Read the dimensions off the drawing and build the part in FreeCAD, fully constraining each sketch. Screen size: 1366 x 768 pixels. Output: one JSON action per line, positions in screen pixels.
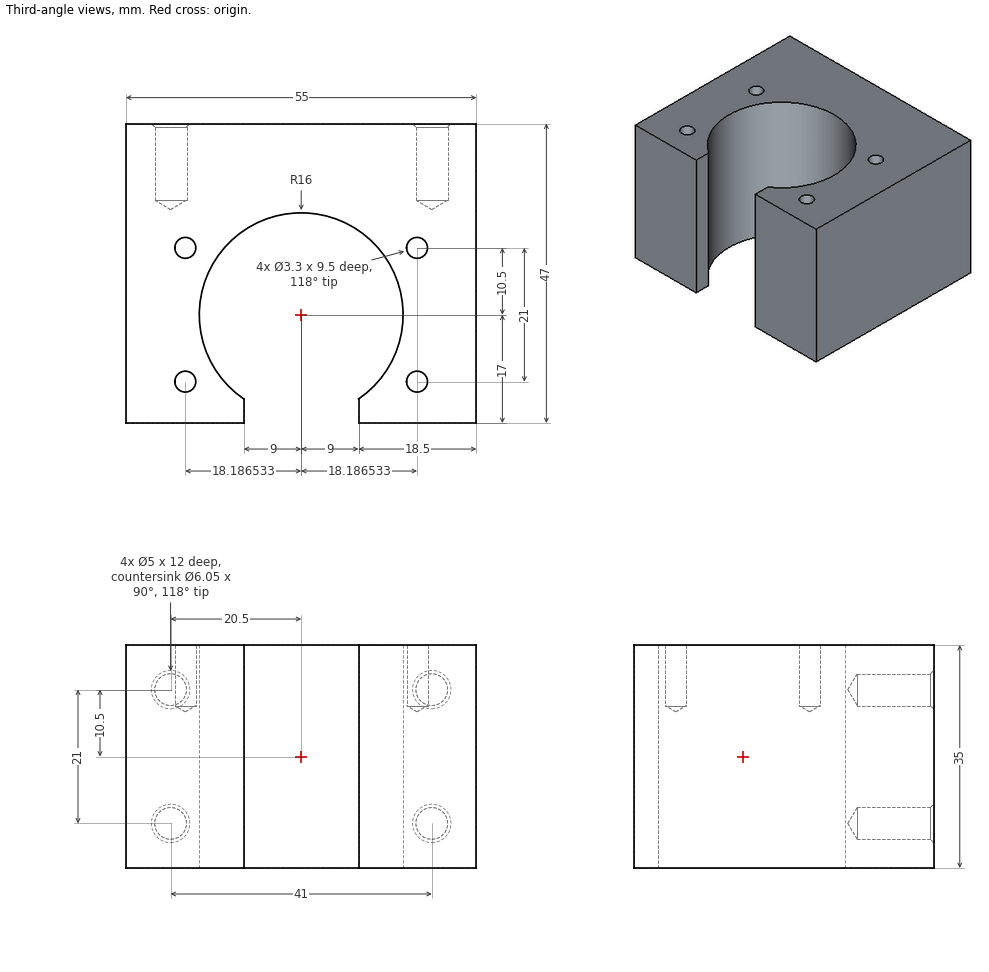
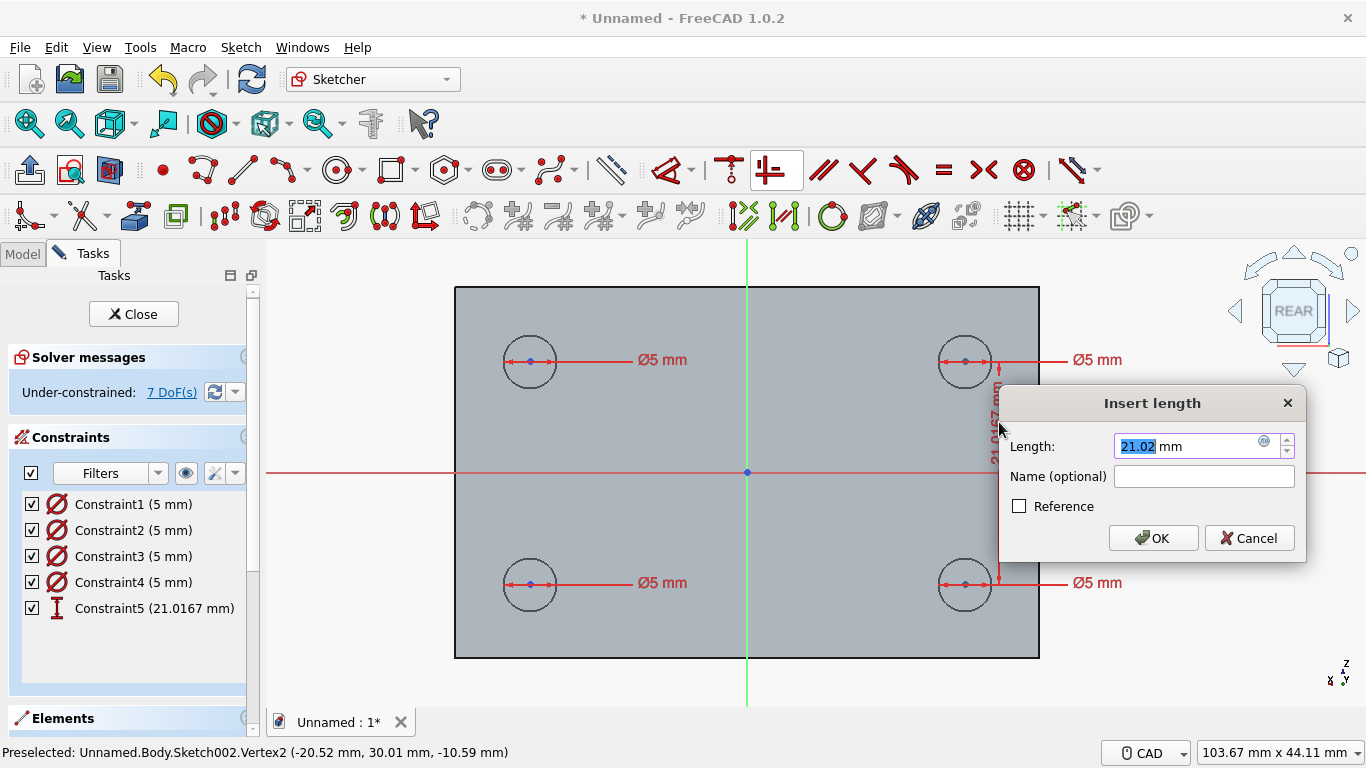
{"action": "type", "text": "21"}
{"action": "key", "text": "Return"}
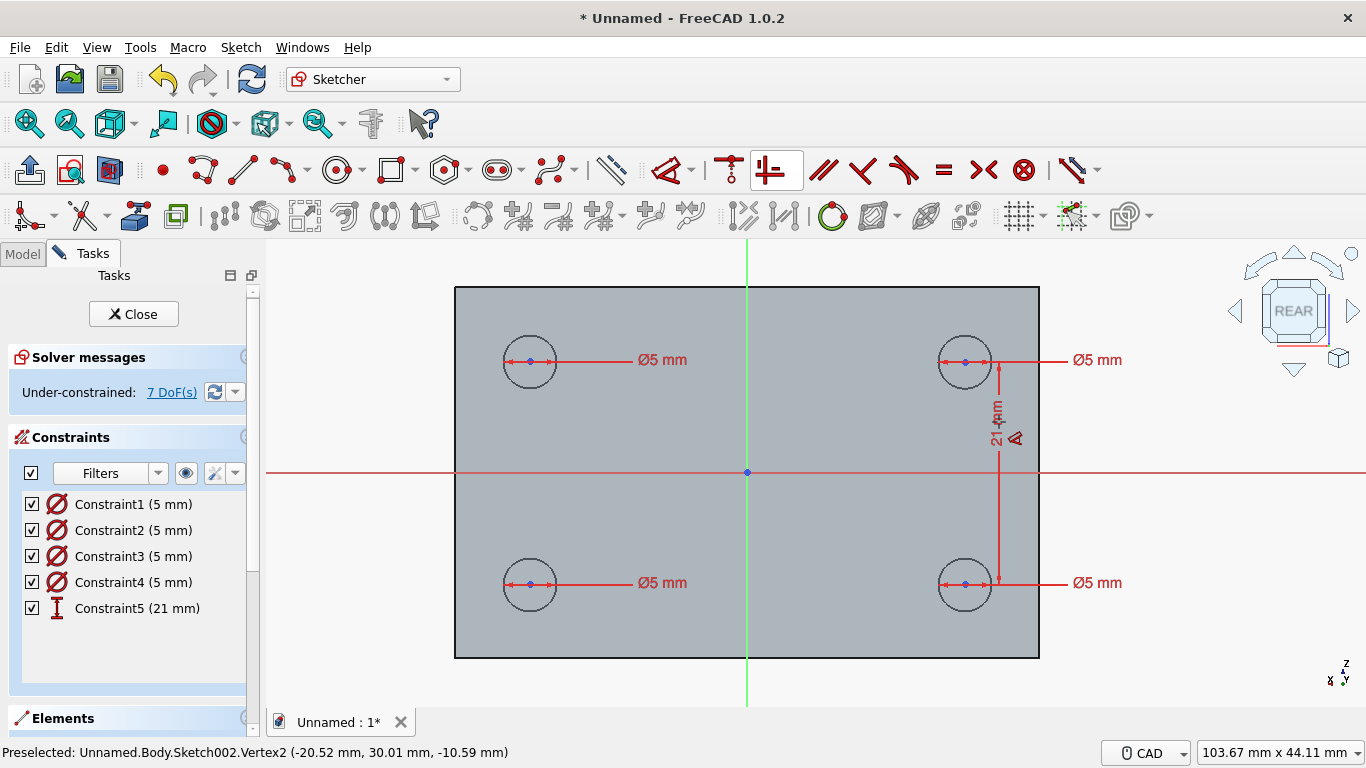
{"action": "left_click", "coordinate": [965, 585]}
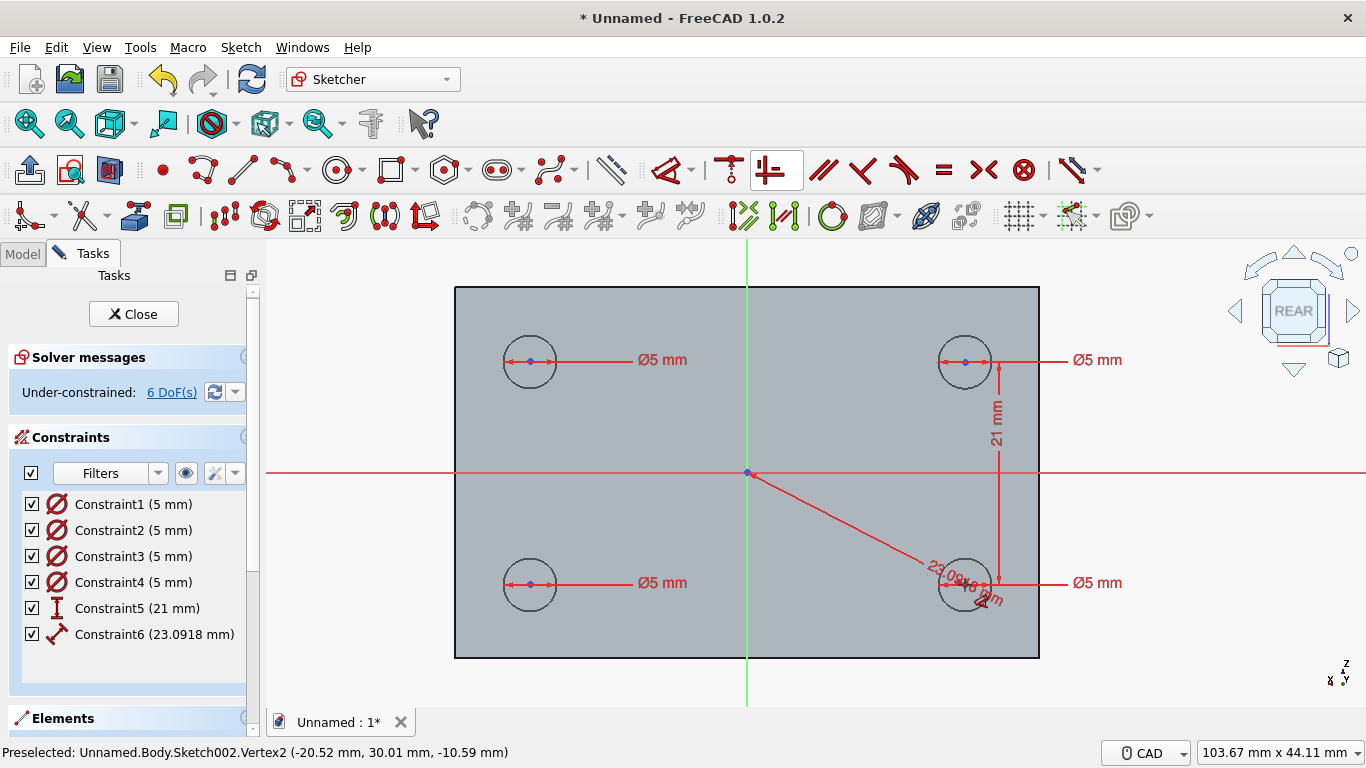
{"action": "left_click", "coordinate": [530, 585]}
{"action": "left_click", "coordinate": [647, 619]}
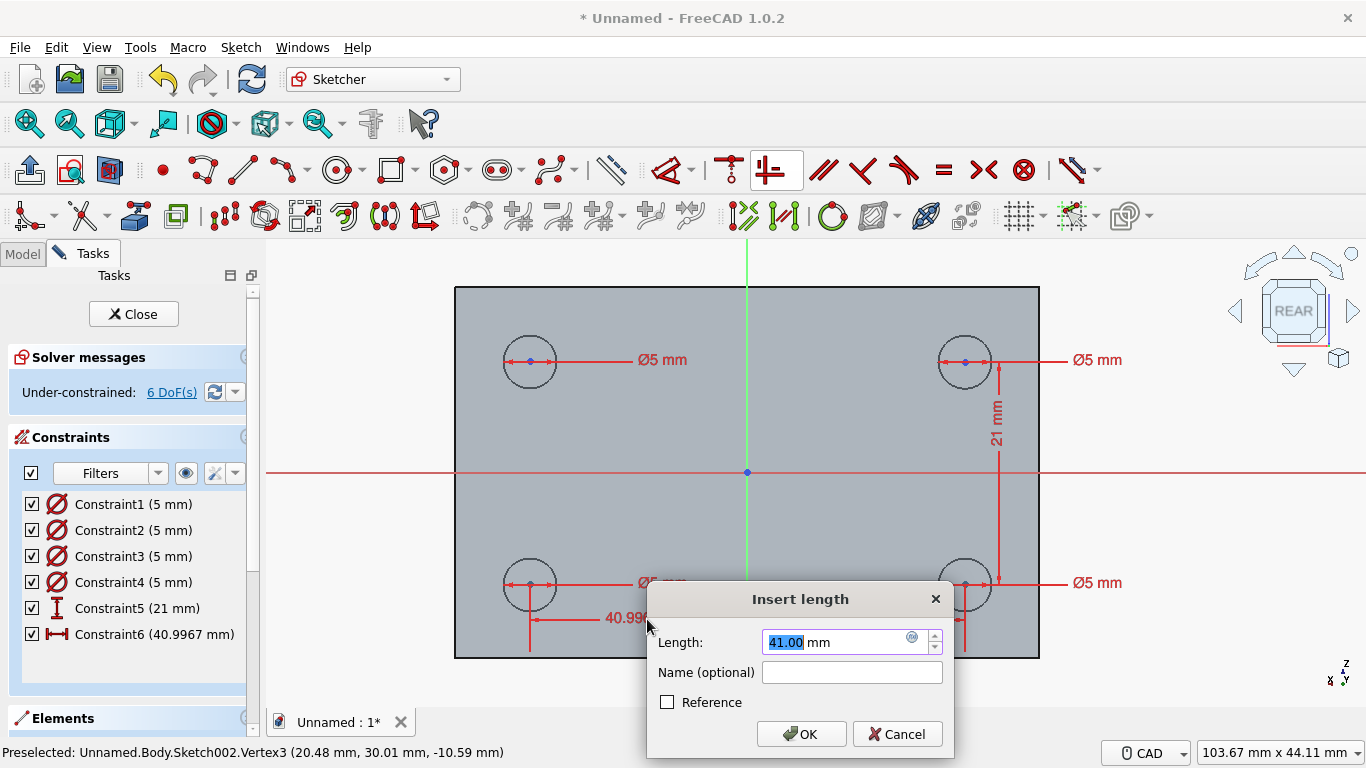
{"action": "type", "text": "41"}
{"action": "key", "text": "Return"}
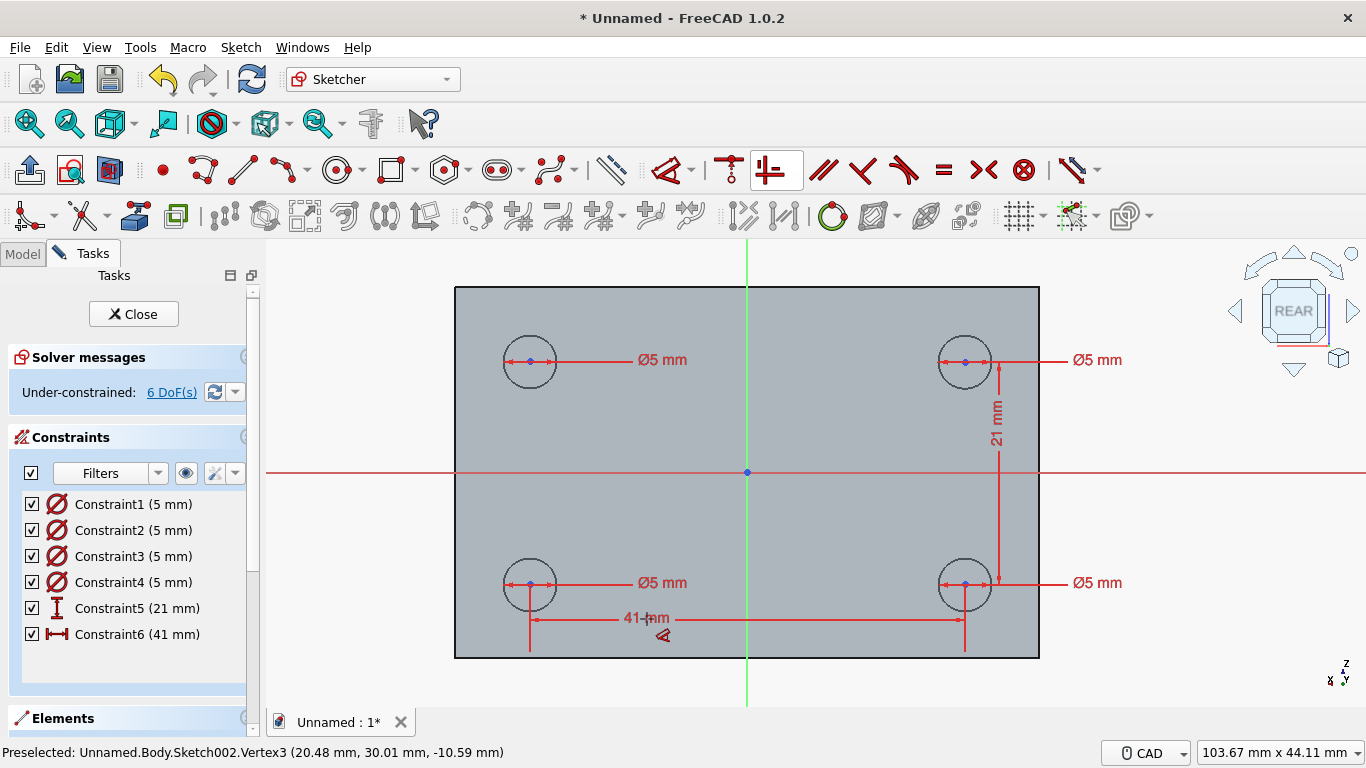
{"action": "left_click", "coordinate": [965, 362]}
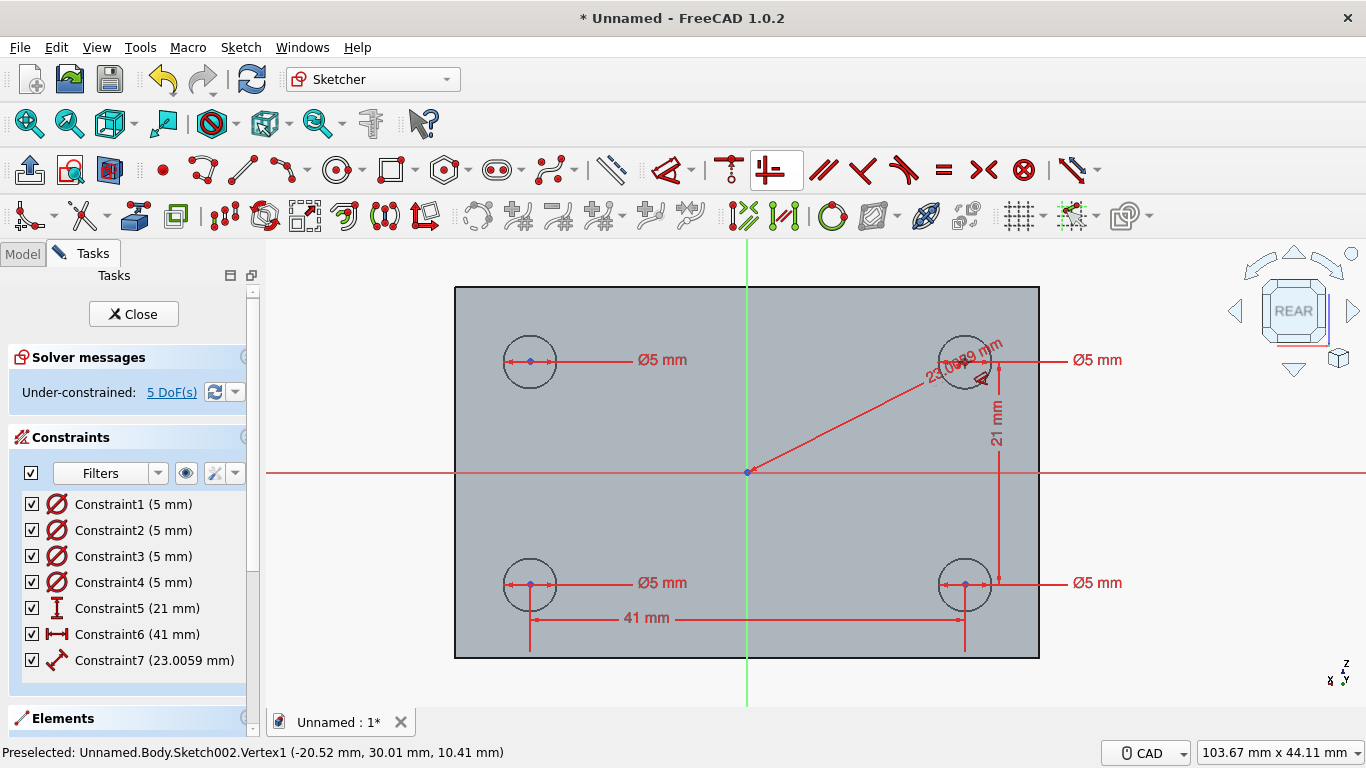
{"action": "left_click", "coordinate": [530, 585]}
{"action": "left_click", "coordinate": [848, 619]}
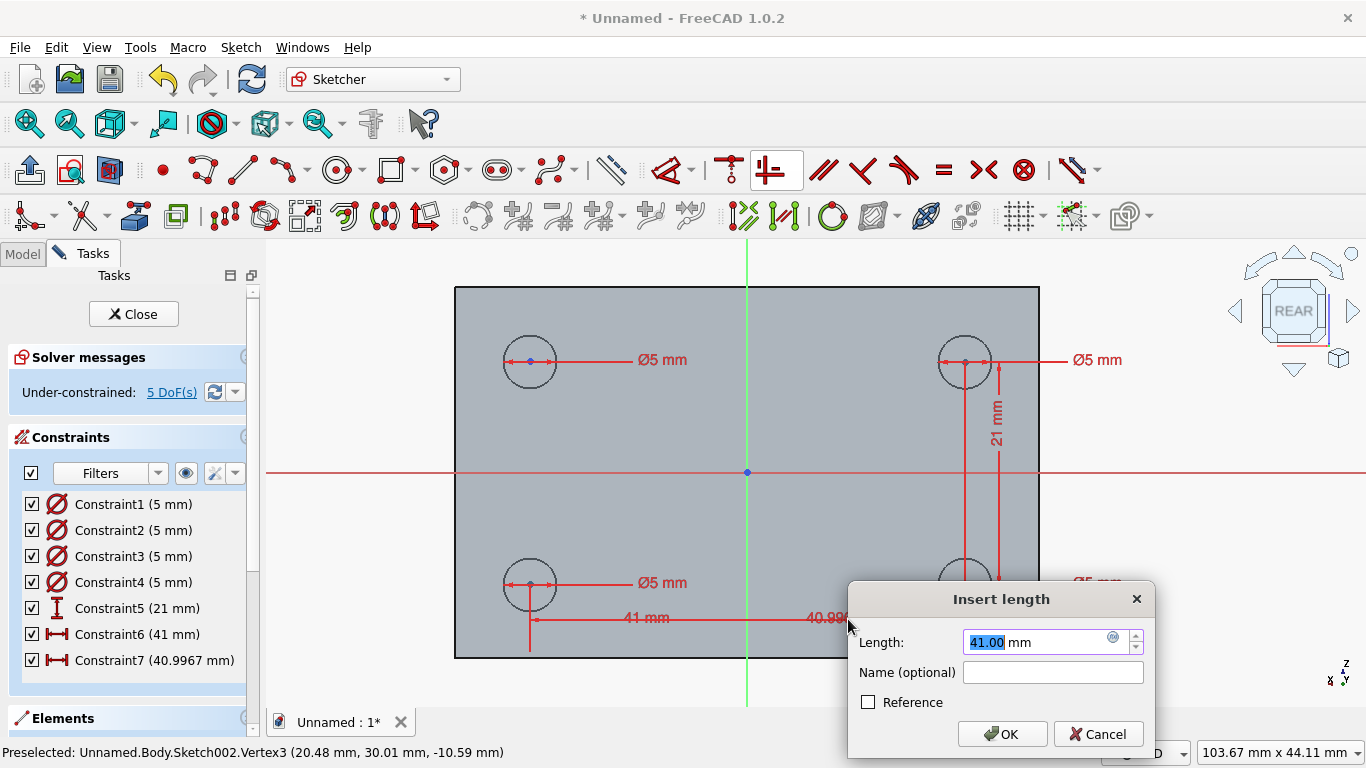
{"action": "type", "text": "41"}
{"action": "key", "text": "Return"}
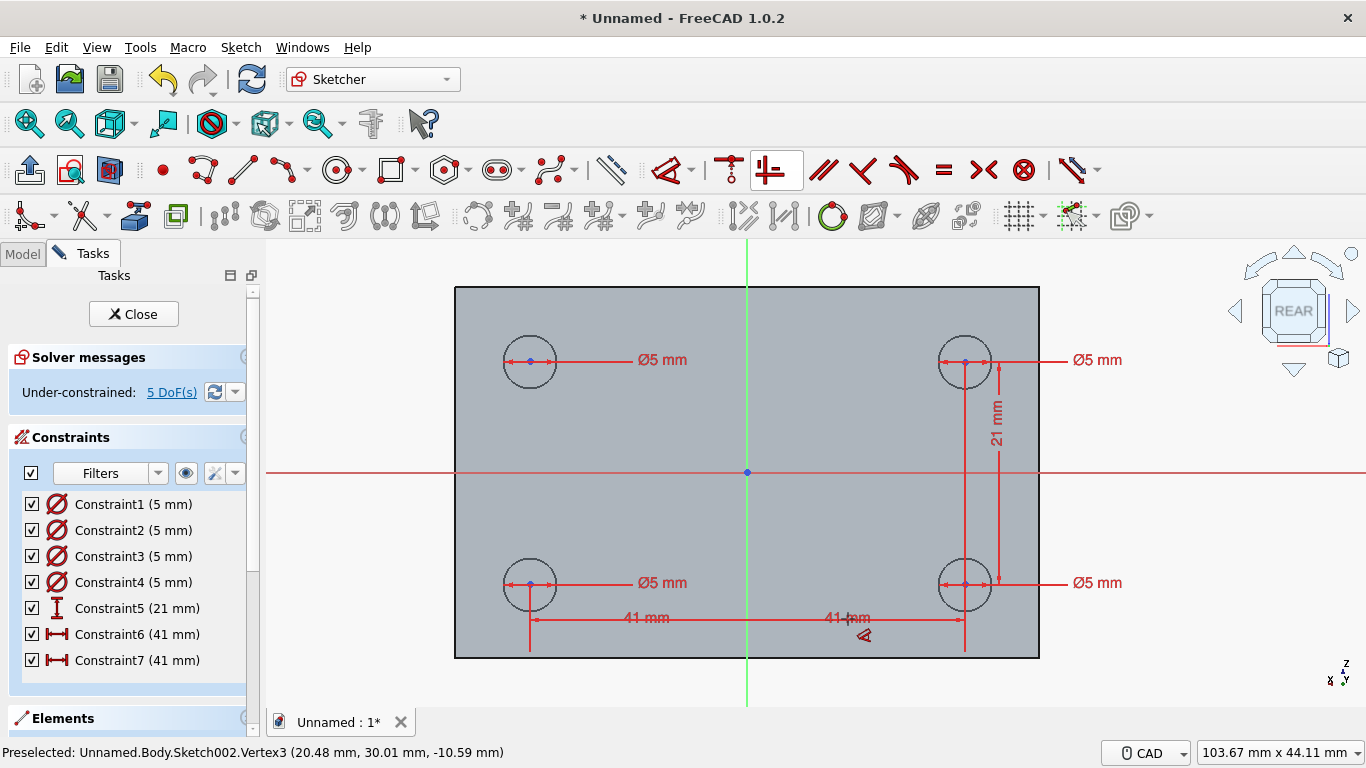
{"action": "left_click", "coordinate": [965, 362]}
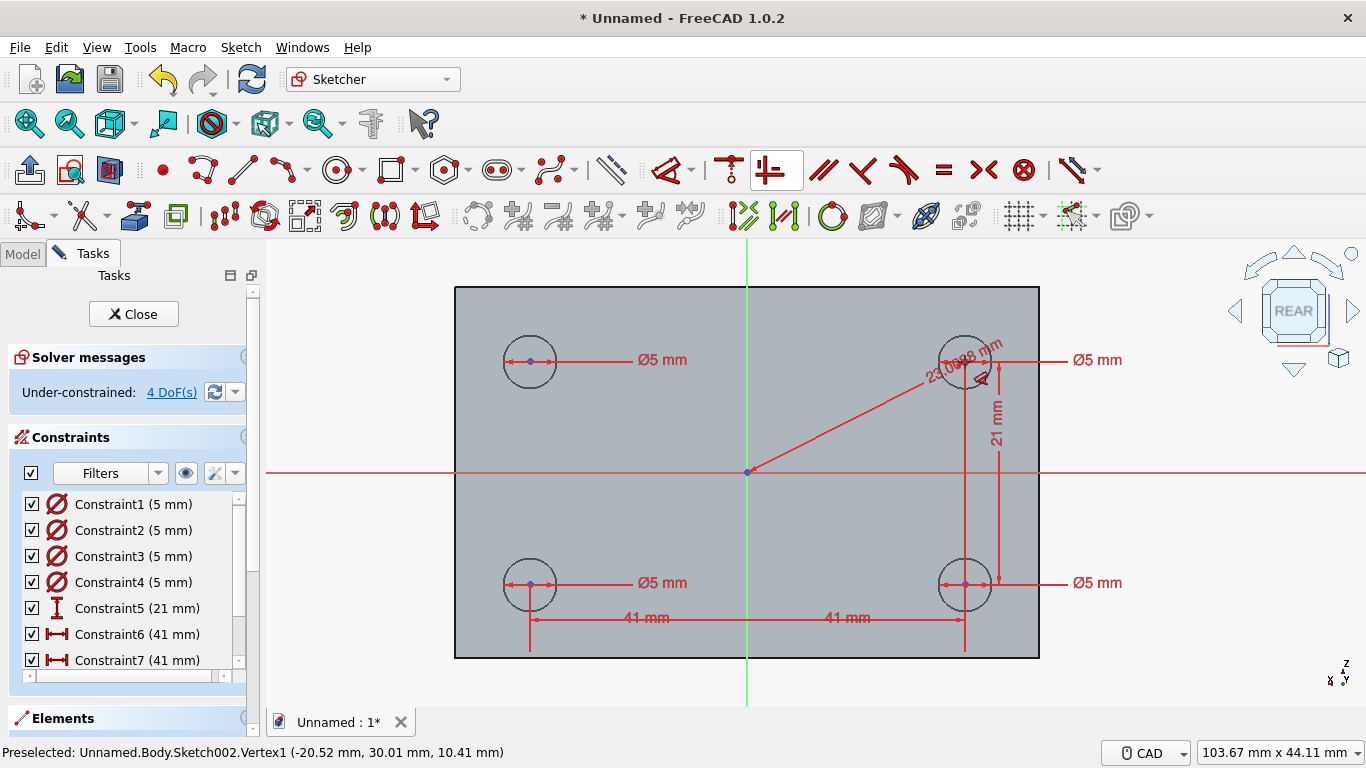
{"action": "left_click", "coordinate": [530, 585]}
{"action": "left_click", "coordinate": [999, 525]}